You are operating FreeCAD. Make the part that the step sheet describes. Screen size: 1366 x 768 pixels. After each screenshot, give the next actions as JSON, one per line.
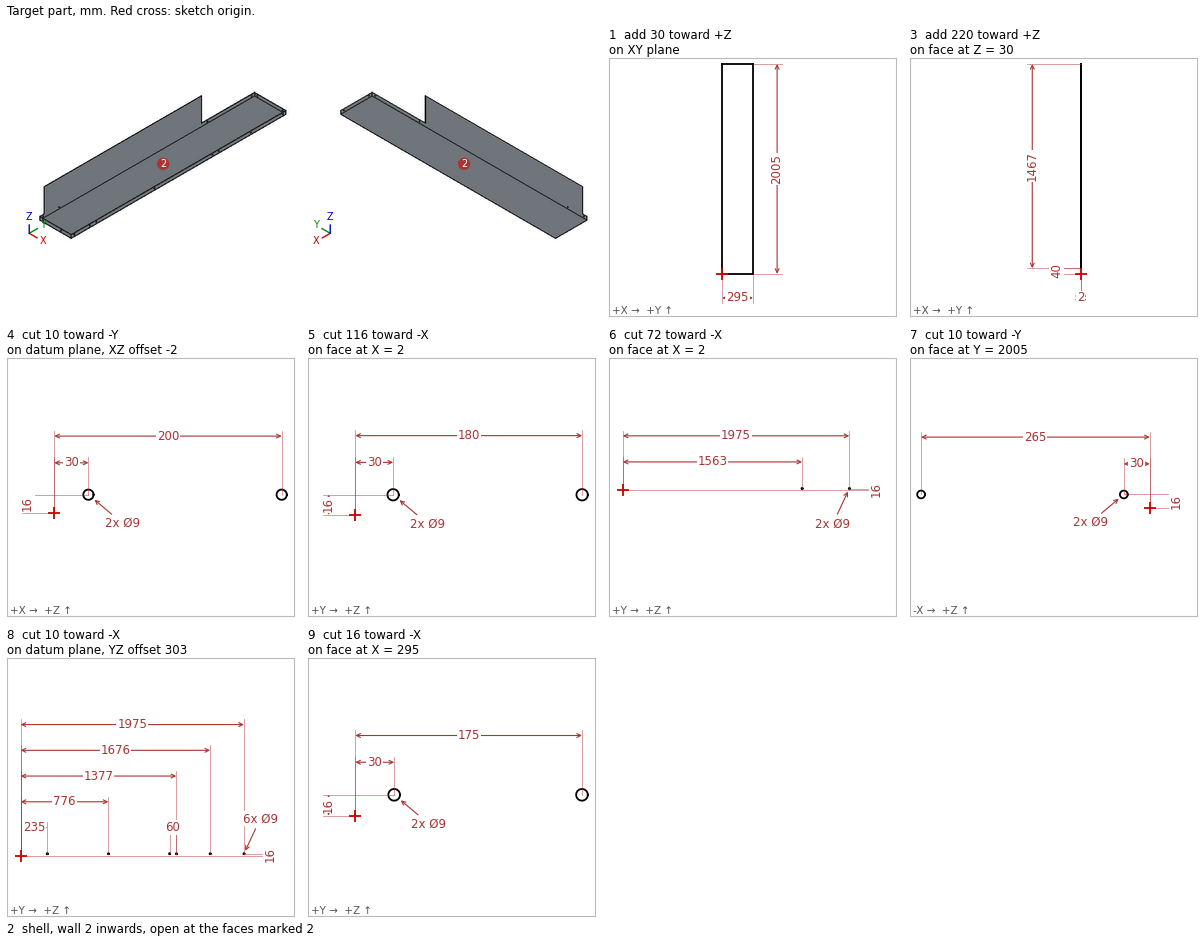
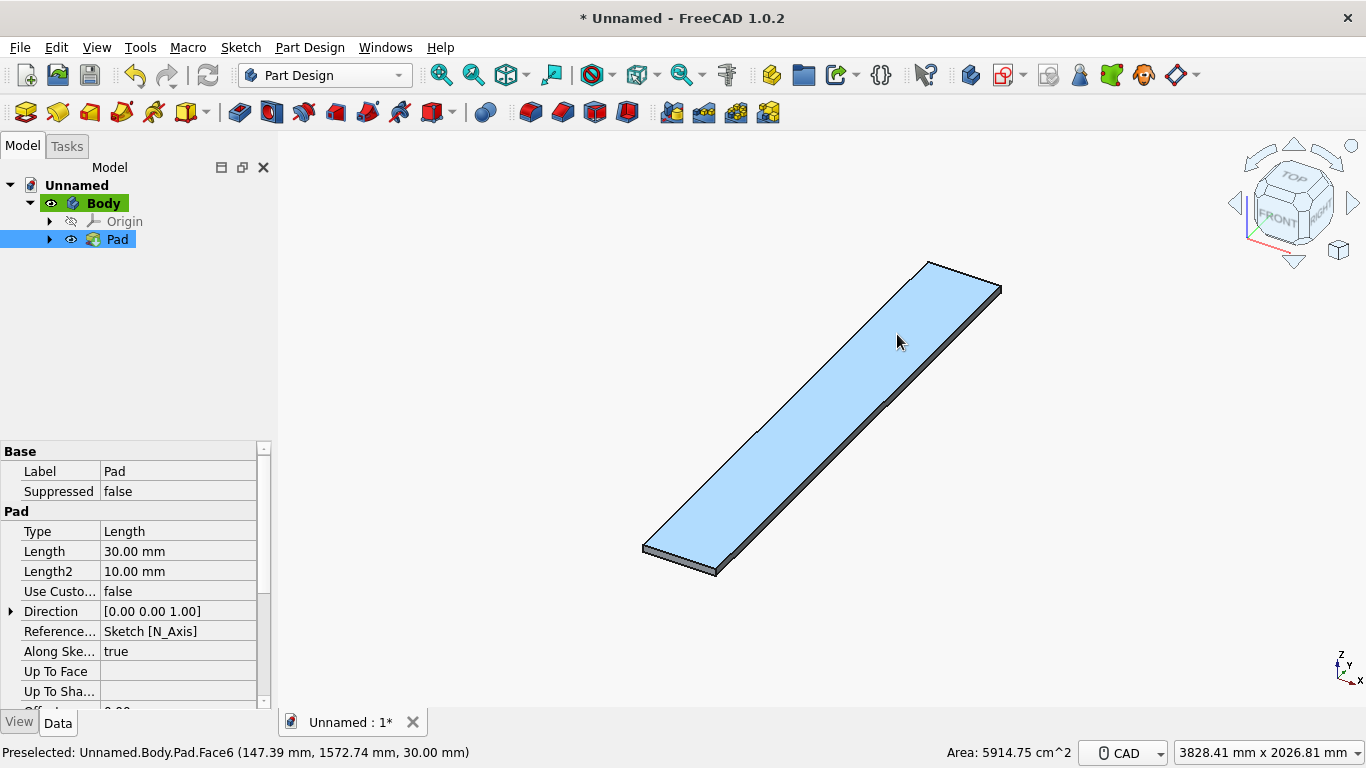
{"action": "left_click", "coordinate": [628, 112]}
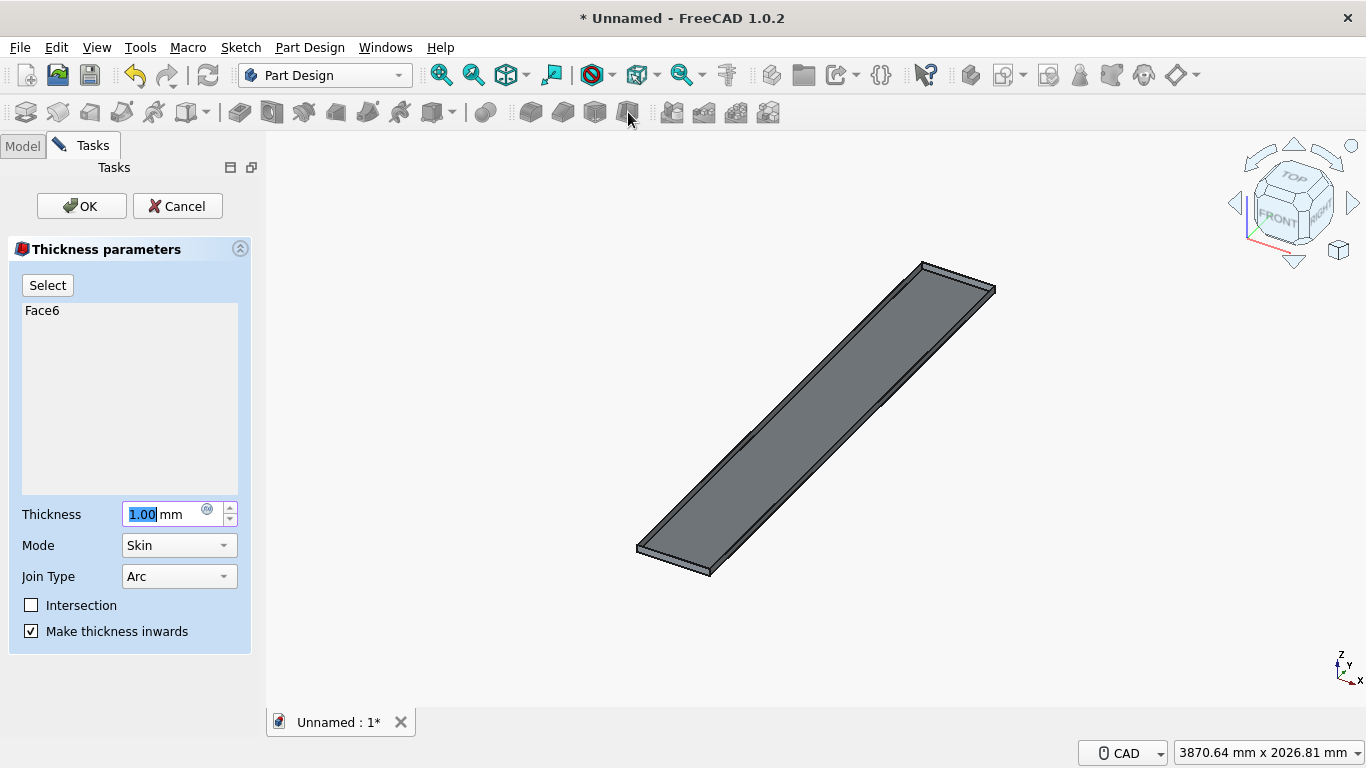
{"action": "type", "text": "2"}
{"action": "key", "text": "Tab"}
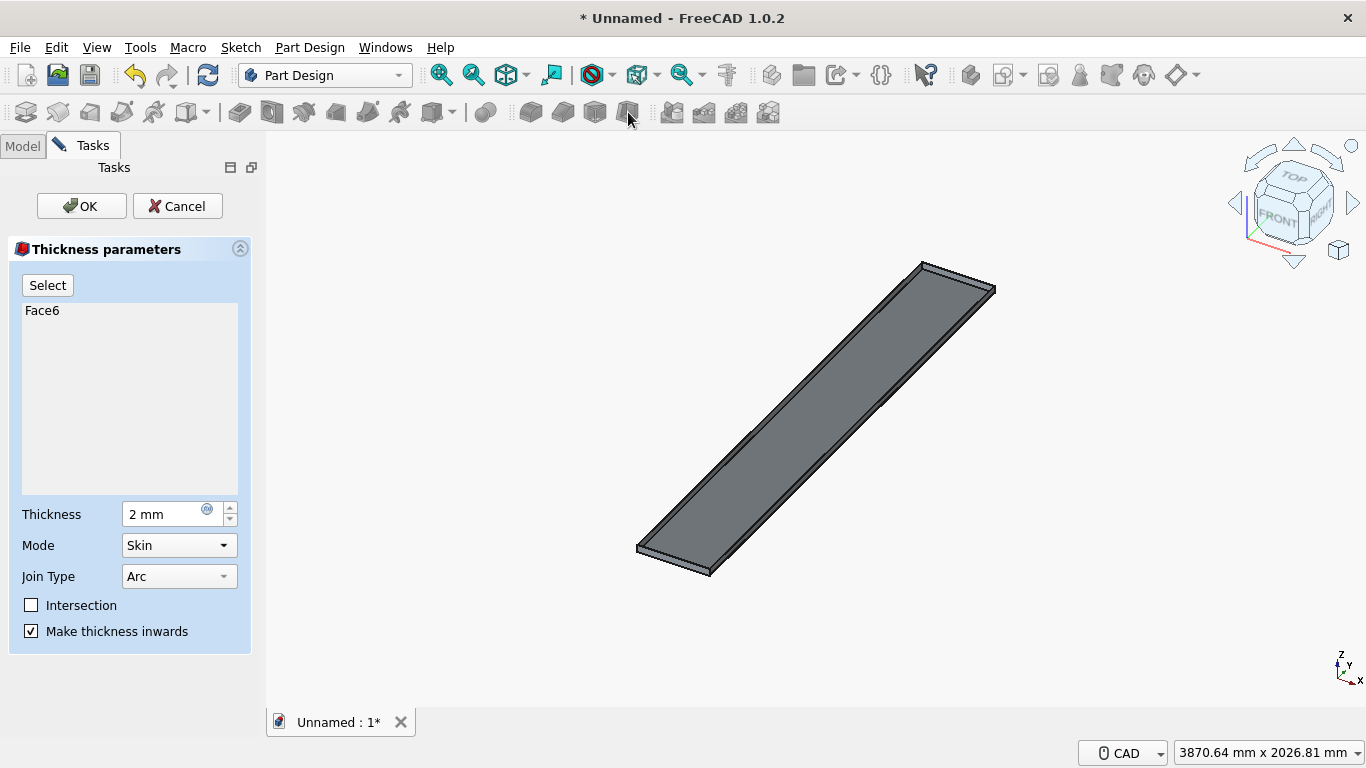
{"action": "left_click", "coordinate": [180, 576]}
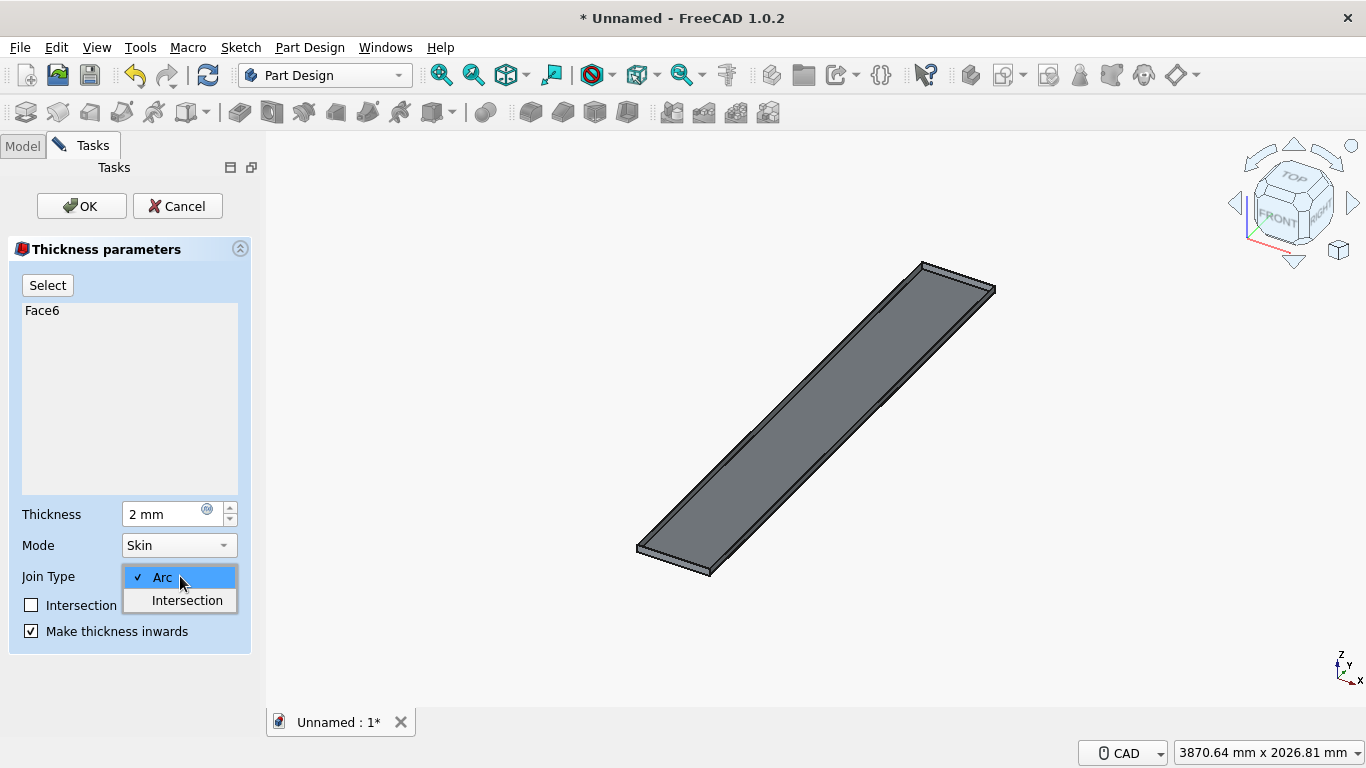
{"action": "left_click", "coordinate": [179, 600]}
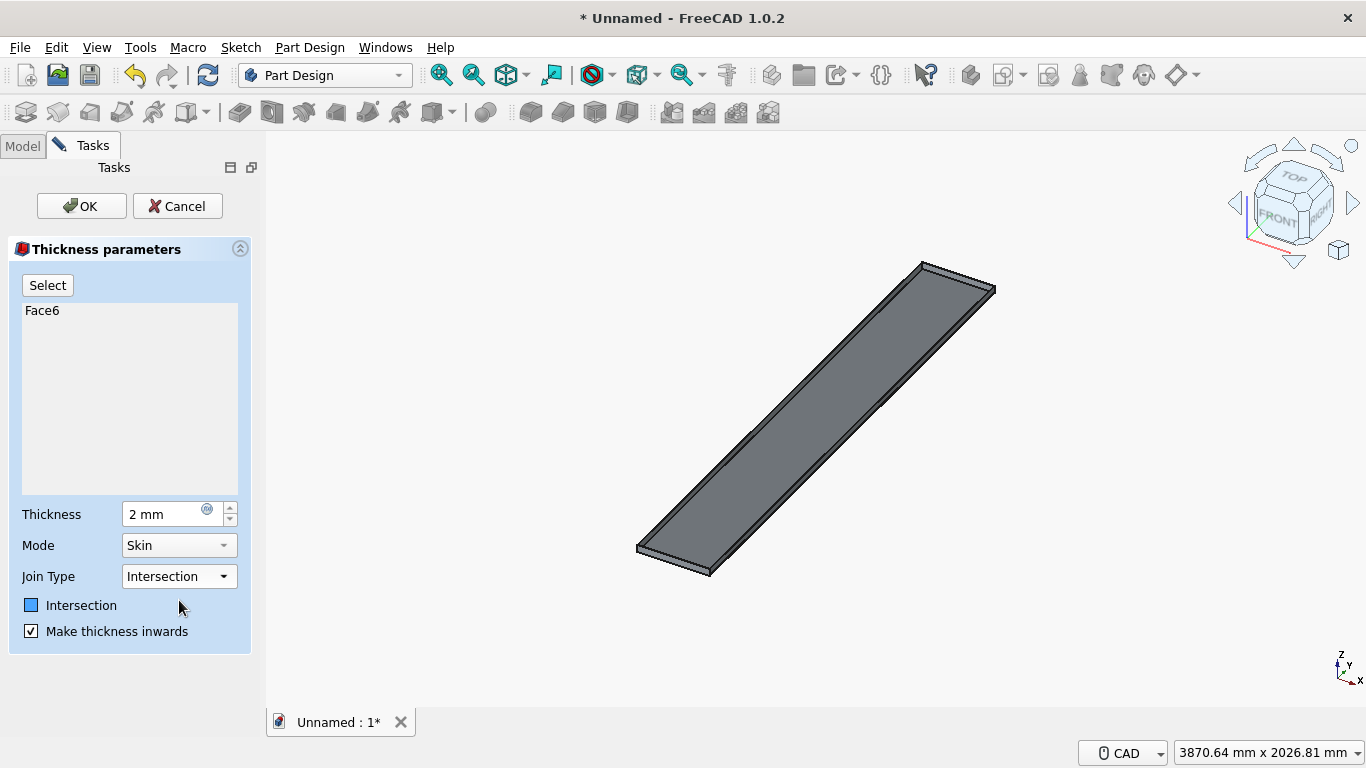
{"action": "left_click", "coordinate": [82, 206]}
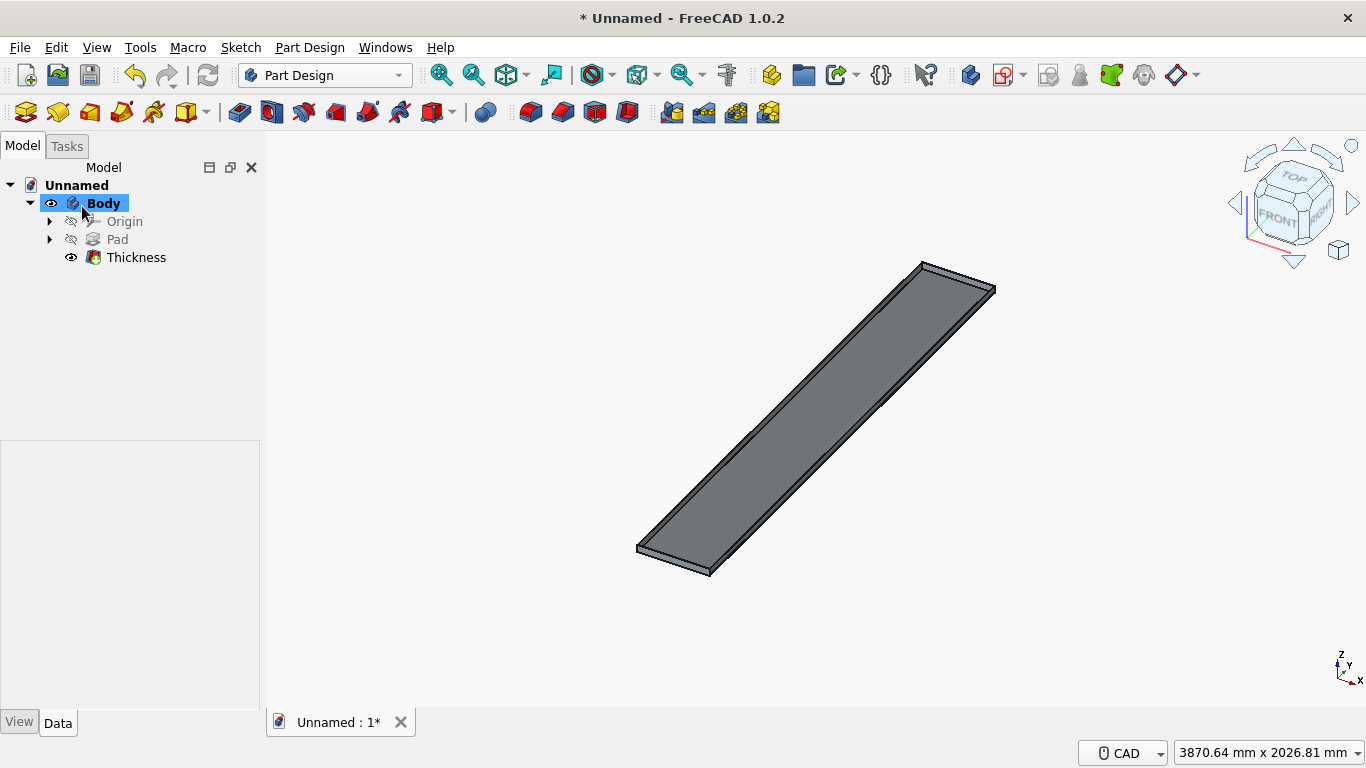
{"action": "scroll", "coordinate": [970, 277], "scroll_direction": "up", "scroll_amount": 15}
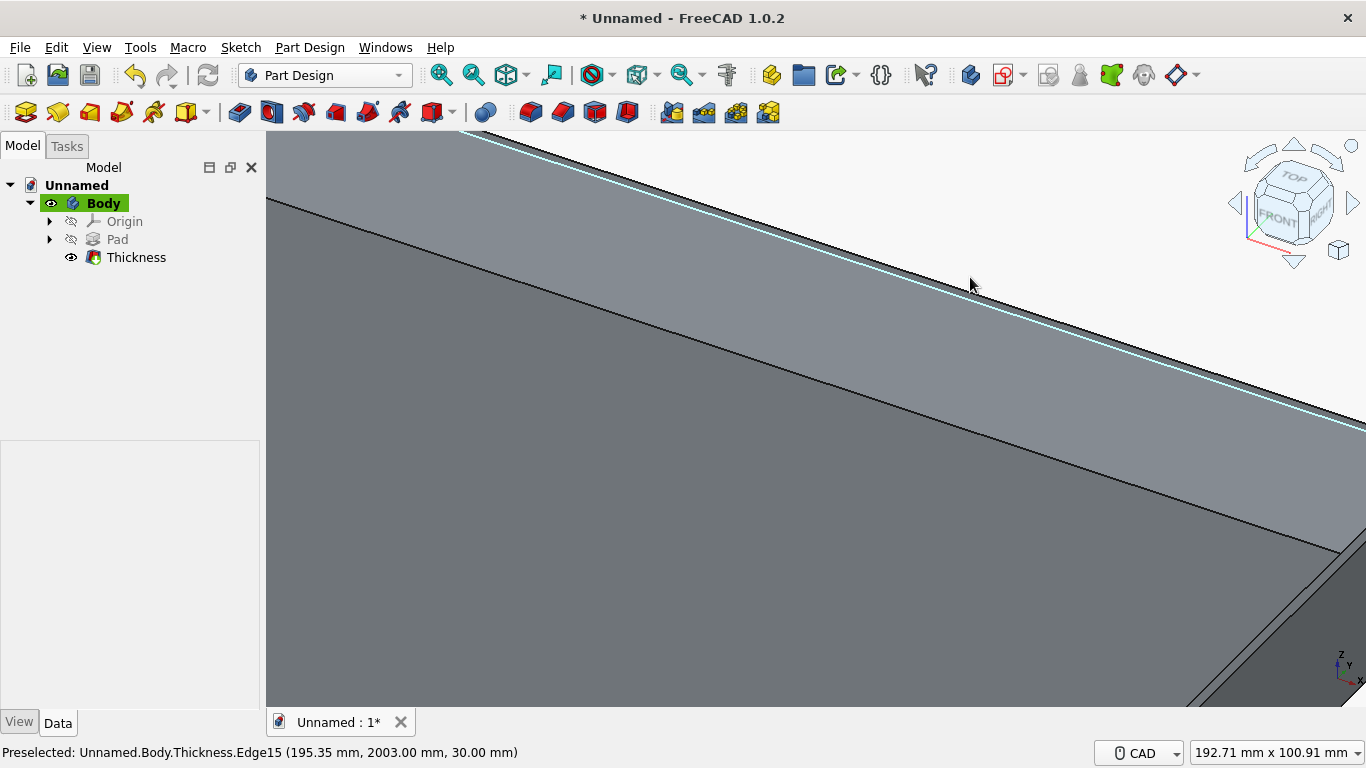
{"action": "scroll", "coordinate": [964, 292], "scroll_direction": "up", "scroll_amount": 6}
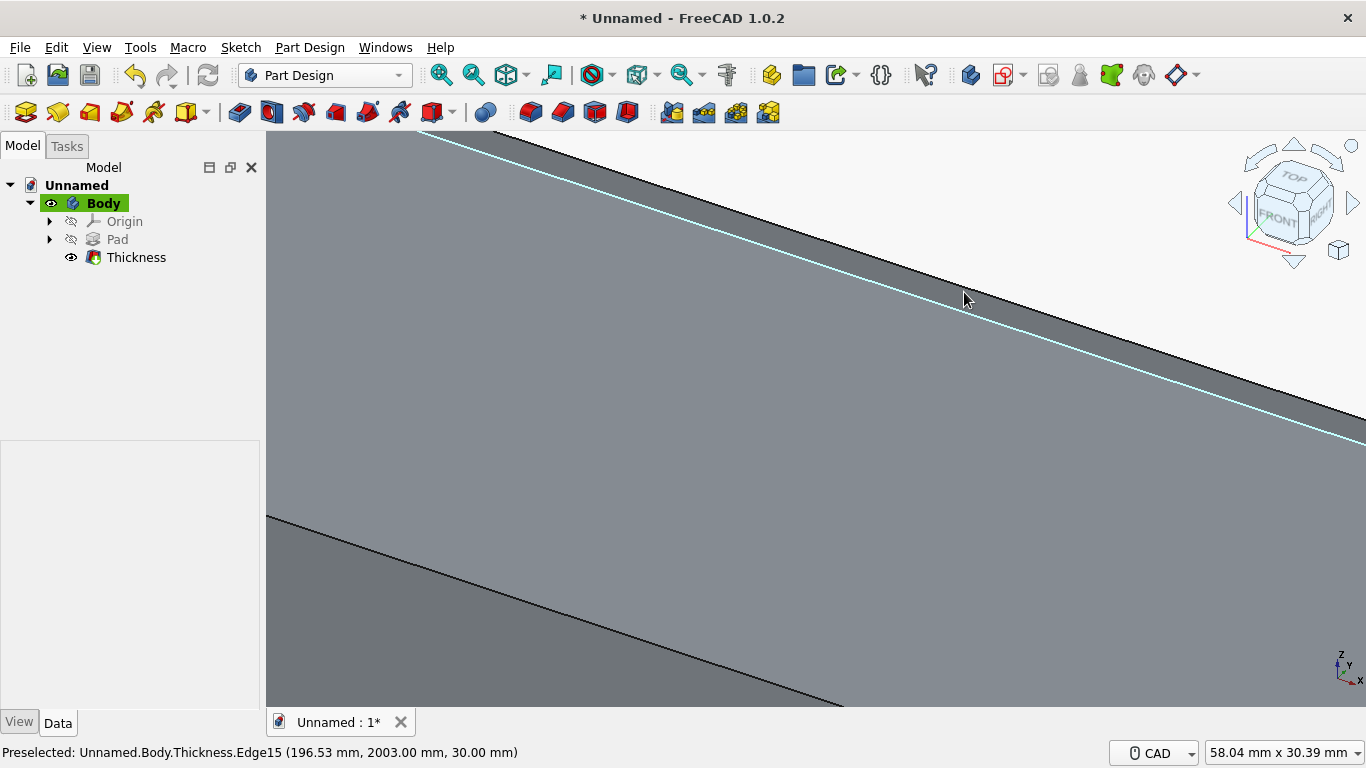
{"action": "left_click", "coordinate": [961, 294]}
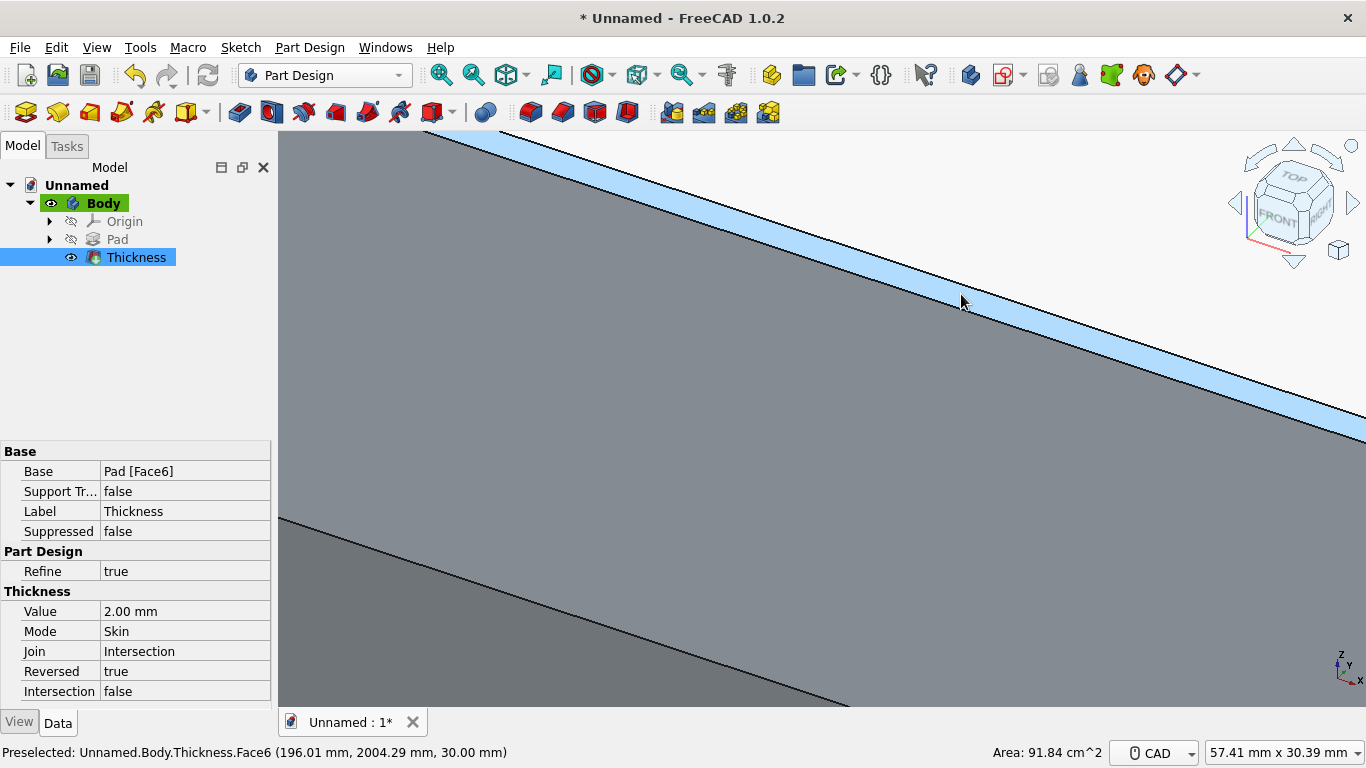
{"action": "left_click", "coordinate": [1004, 76]}